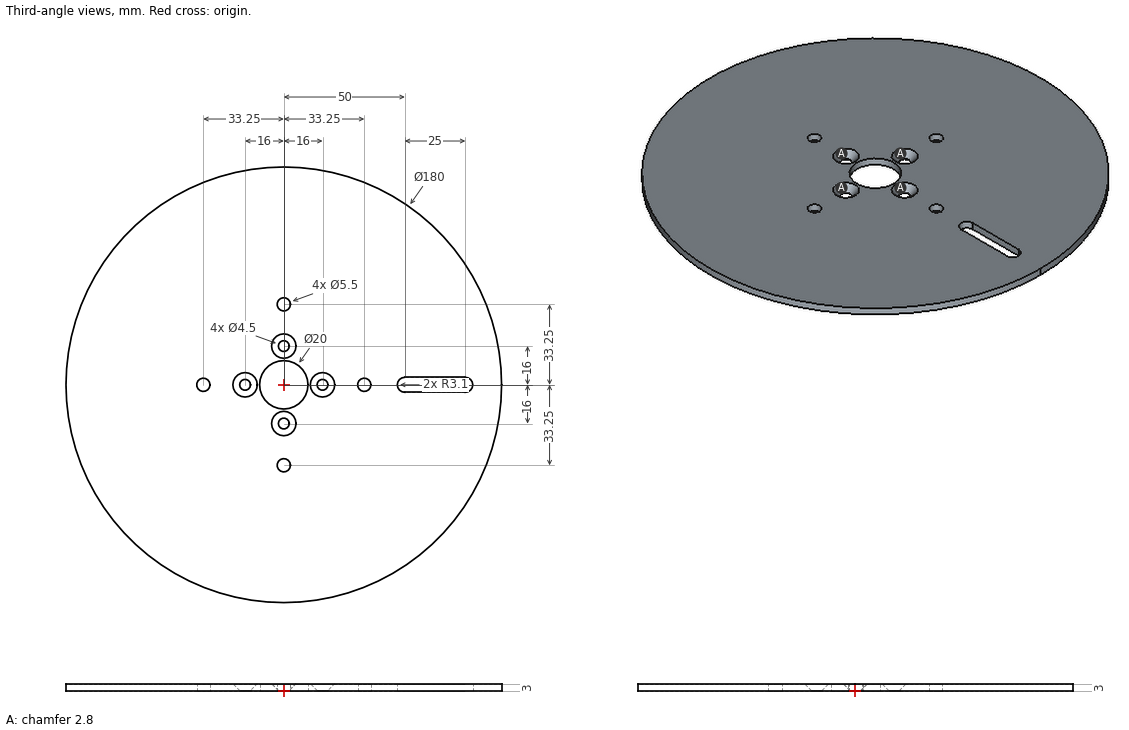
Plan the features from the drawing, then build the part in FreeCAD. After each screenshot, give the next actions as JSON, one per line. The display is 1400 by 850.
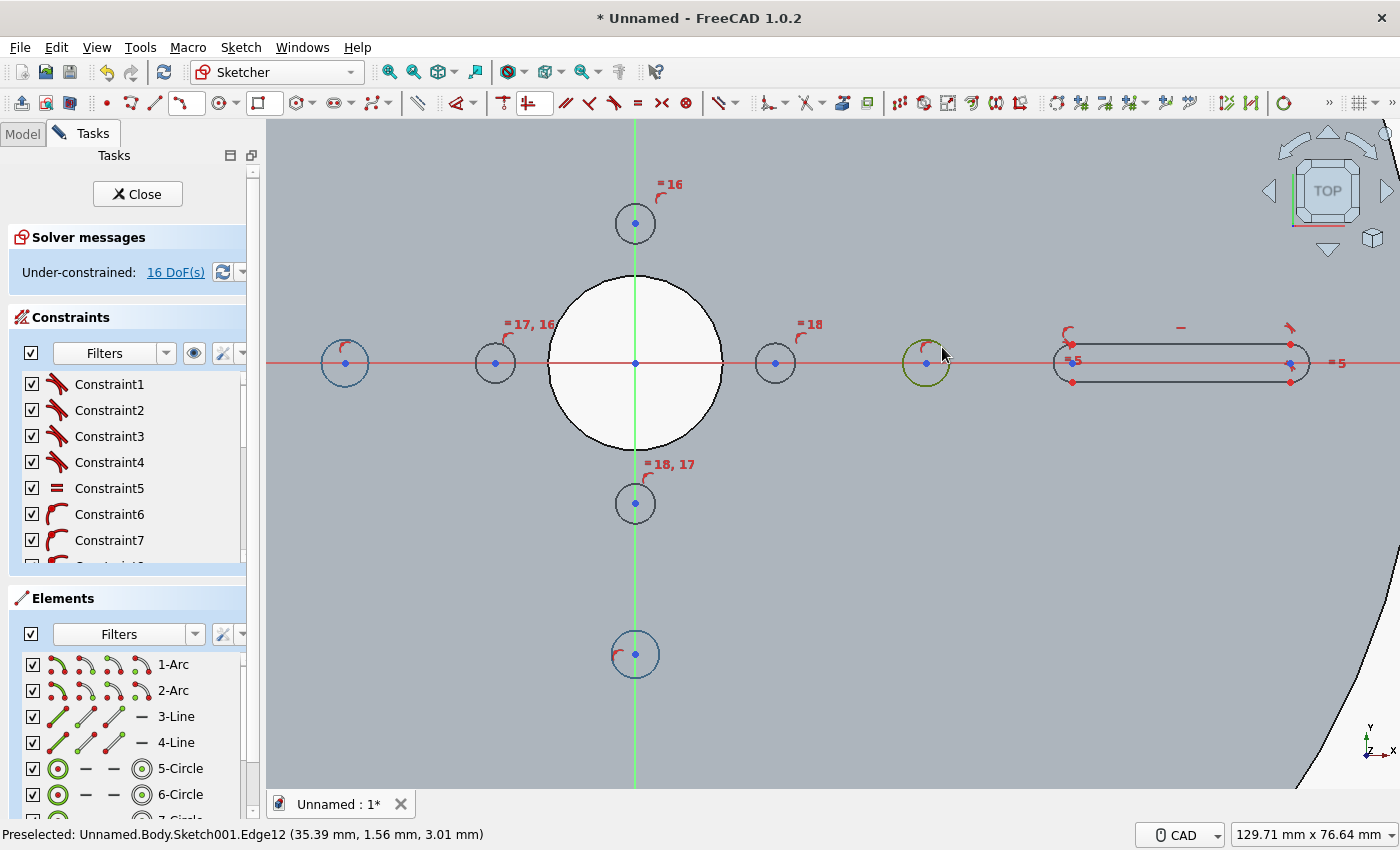
{"action": "left_click", "coordinate": [638, 104]}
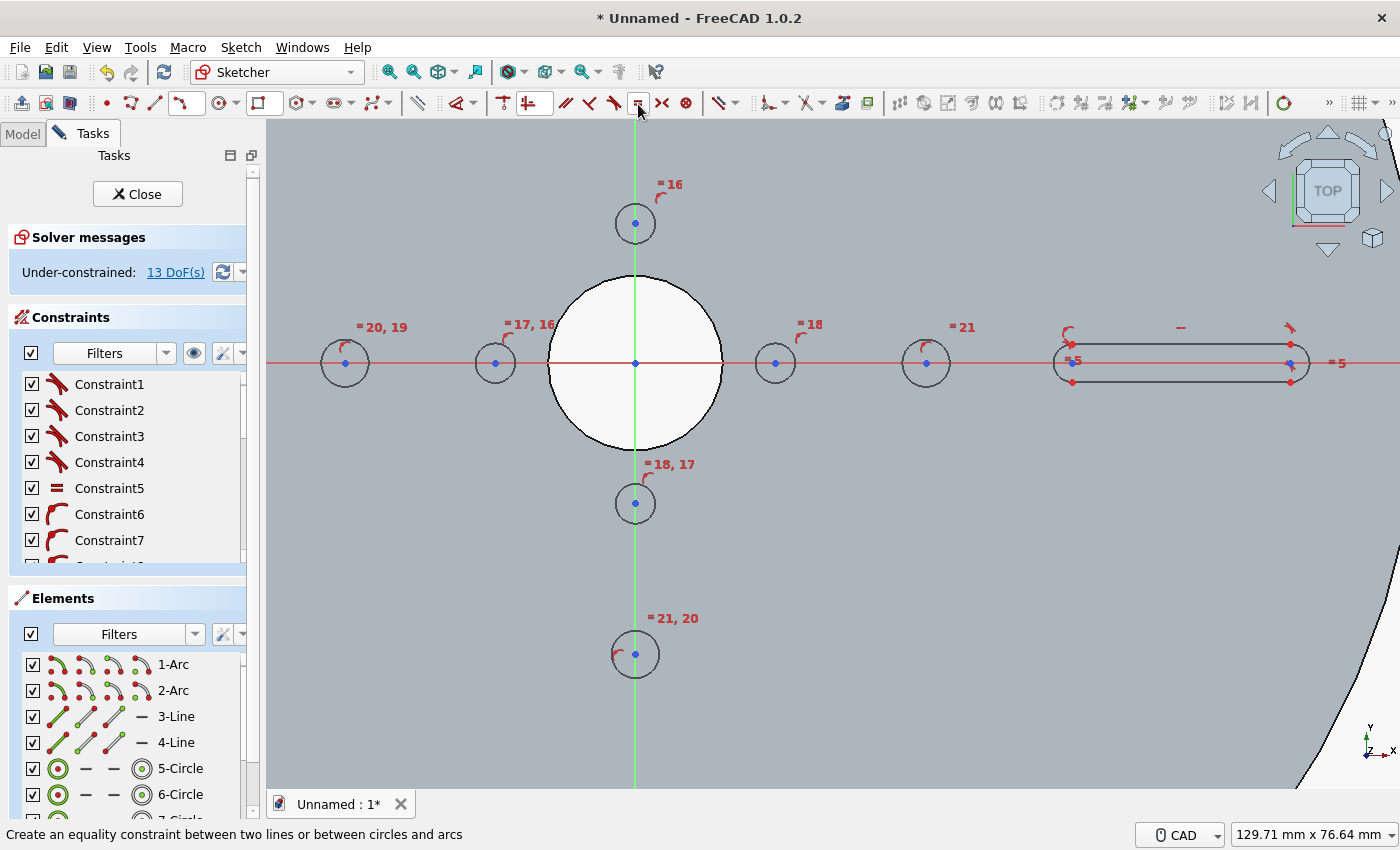
{"action": "left_click", "coordinate": [456, 104]}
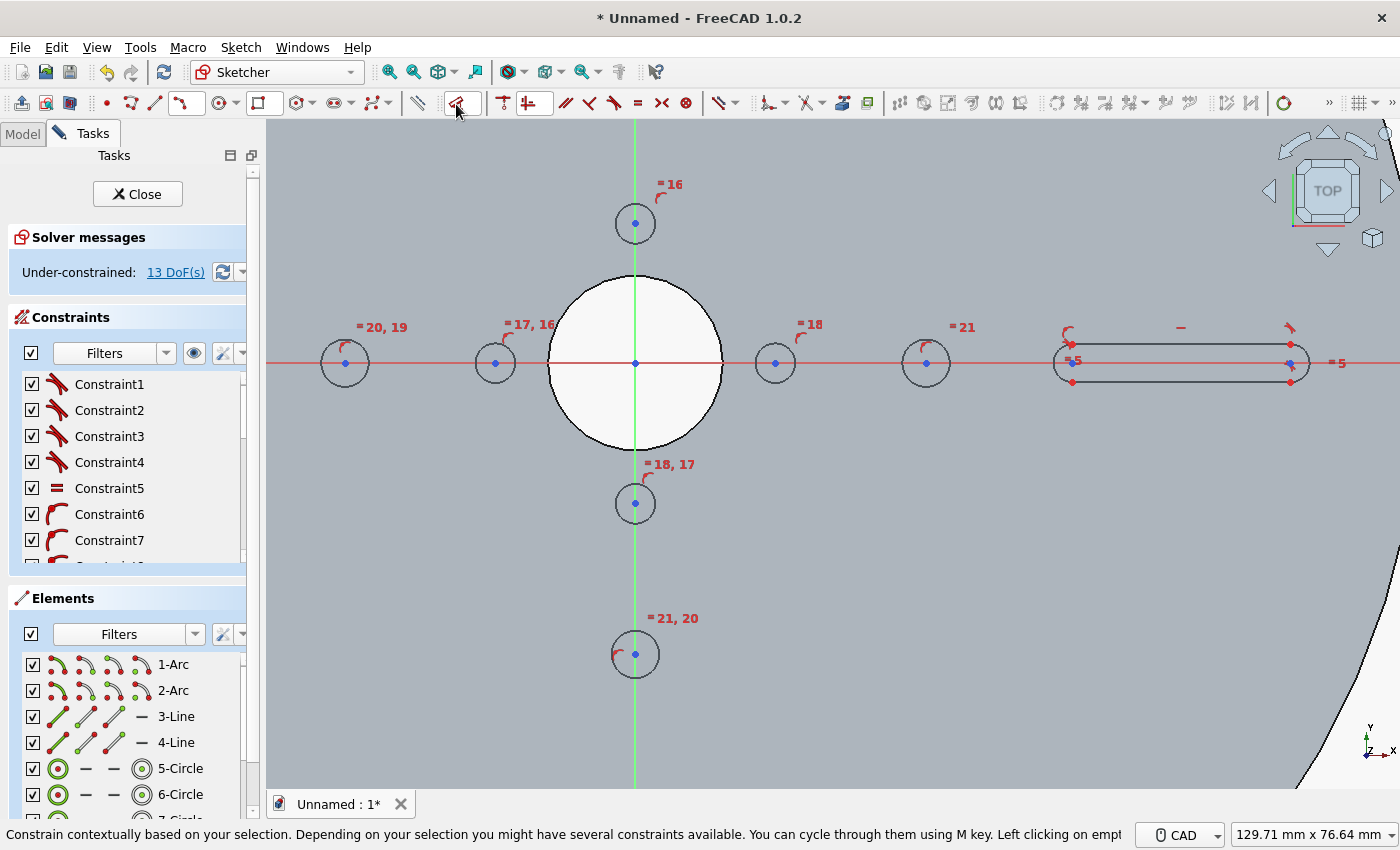
{"action": "scroll", "coordinate": [1057, 352], "scroll_direction": "up", "scroll_amount": 2}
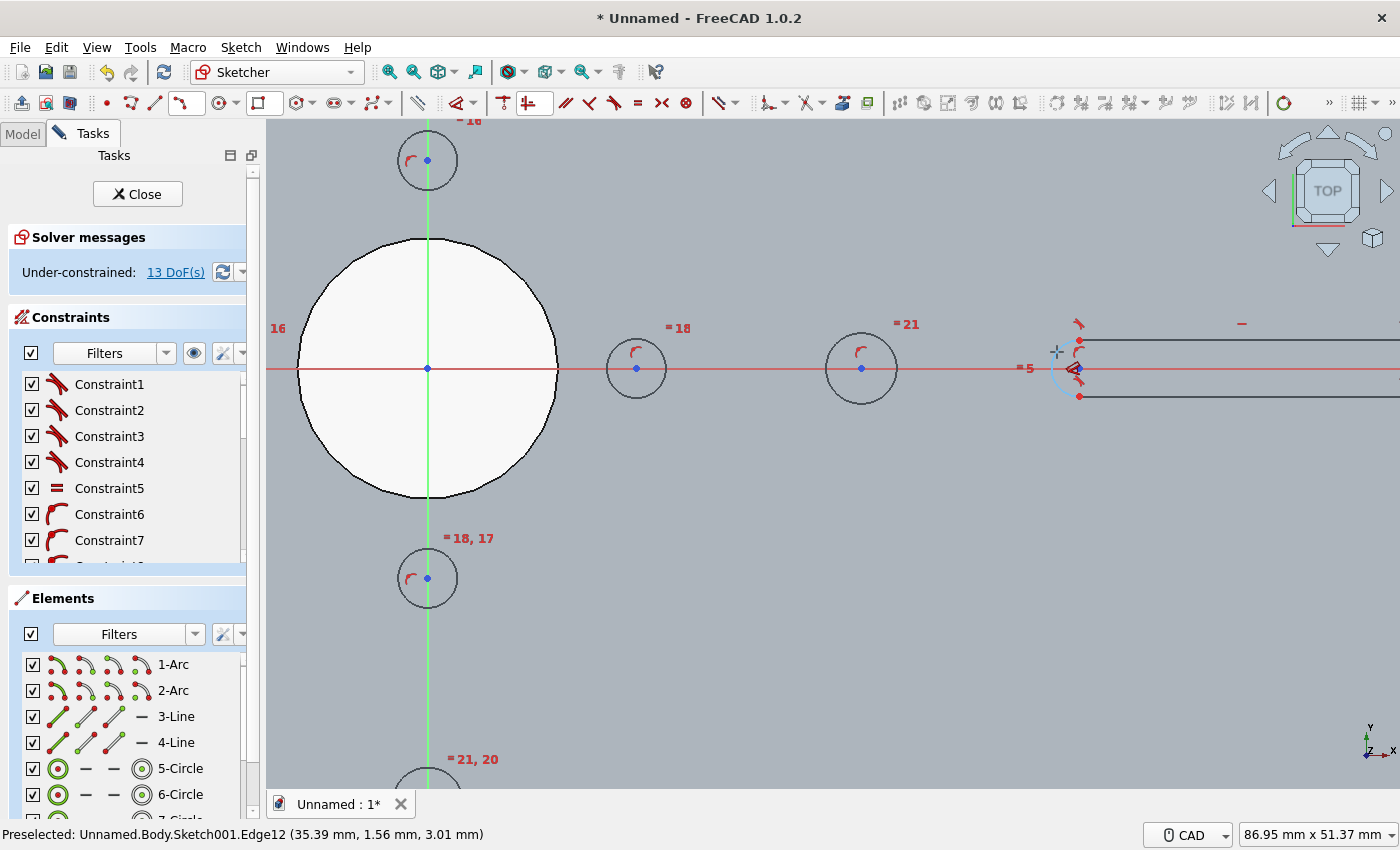
{"action": "left_click", "coordinate": [1057, 352]}
{"action": "left_click", "coordinate": [1031, 333]}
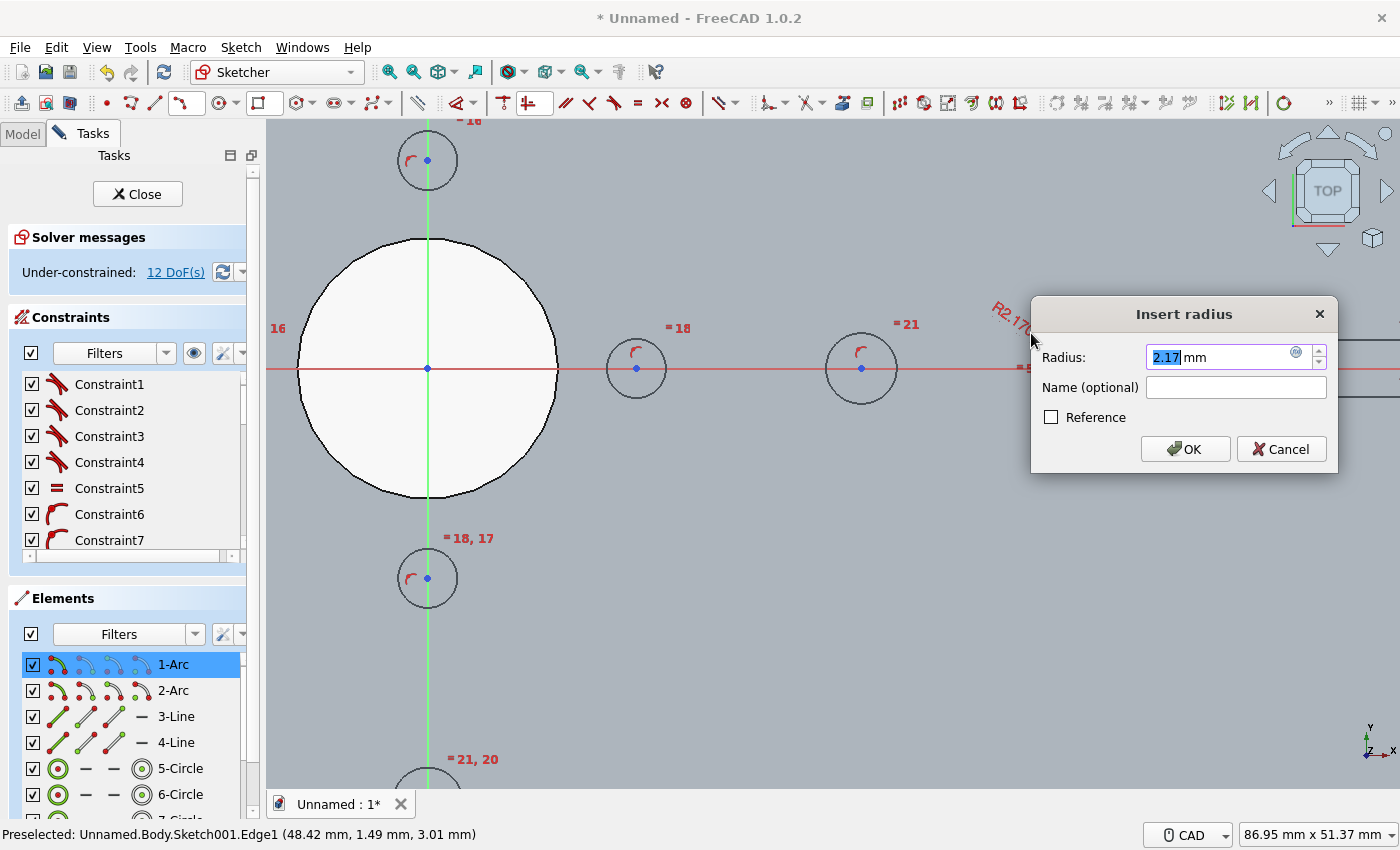
{"action": "type", "text": "3.1"}
{"action": "key", "text": "Return"}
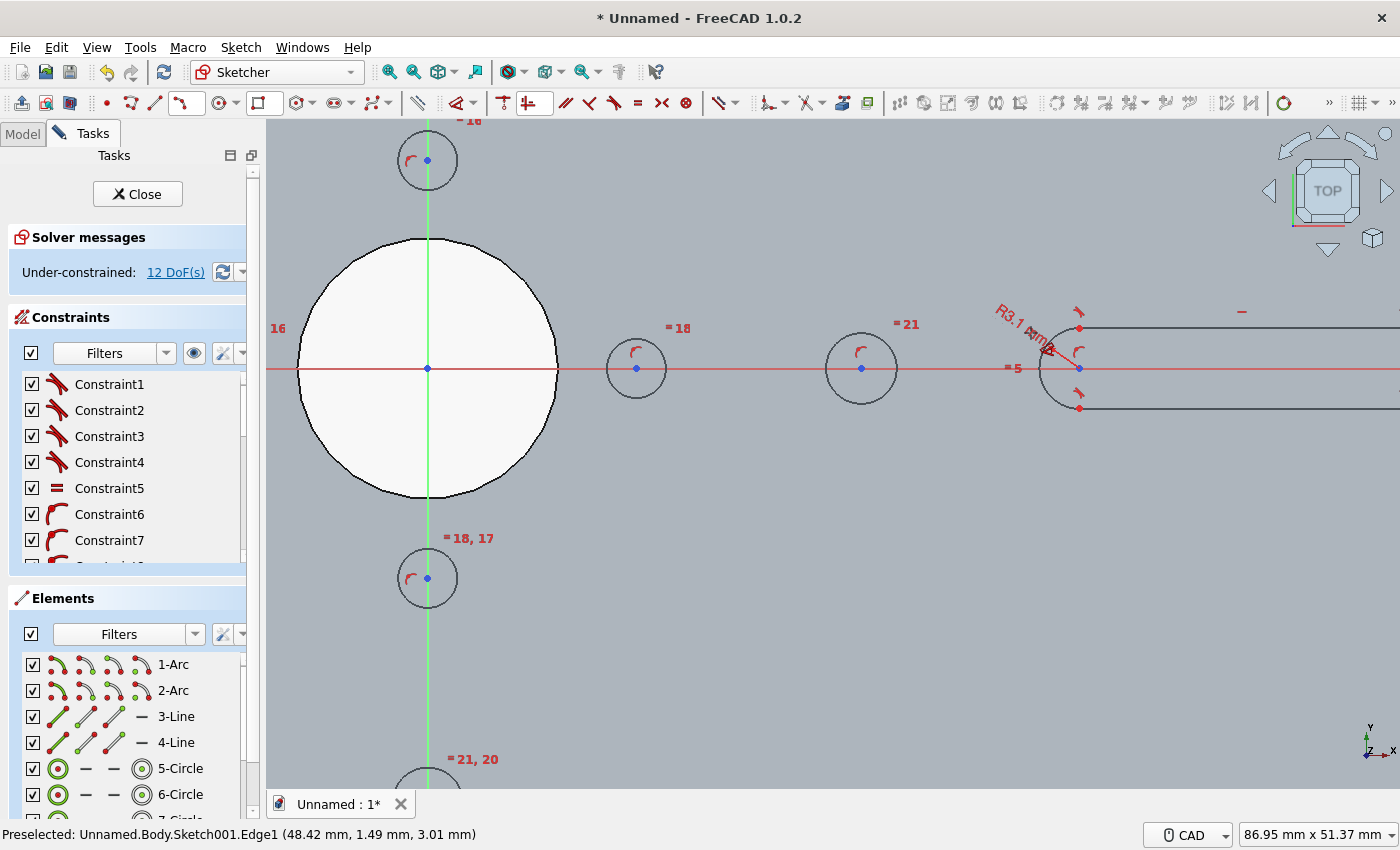
{"action": "left_click", "coordinate": [407, 182]}
{"action": "left_click", "coordinate": [385, 205]}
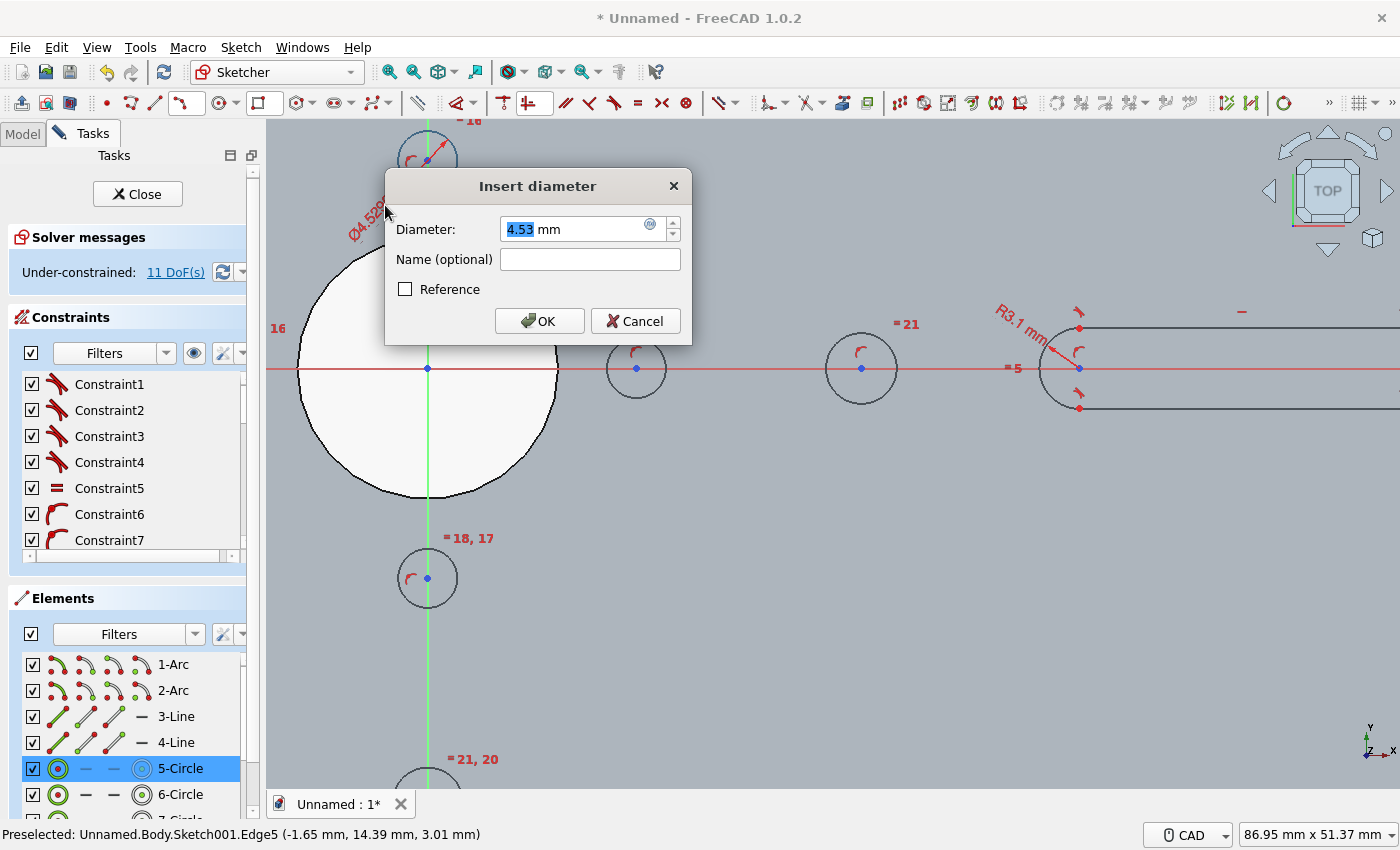
{"action": "type", "text": "4.5"}
{"action": "key", "text": "Return"}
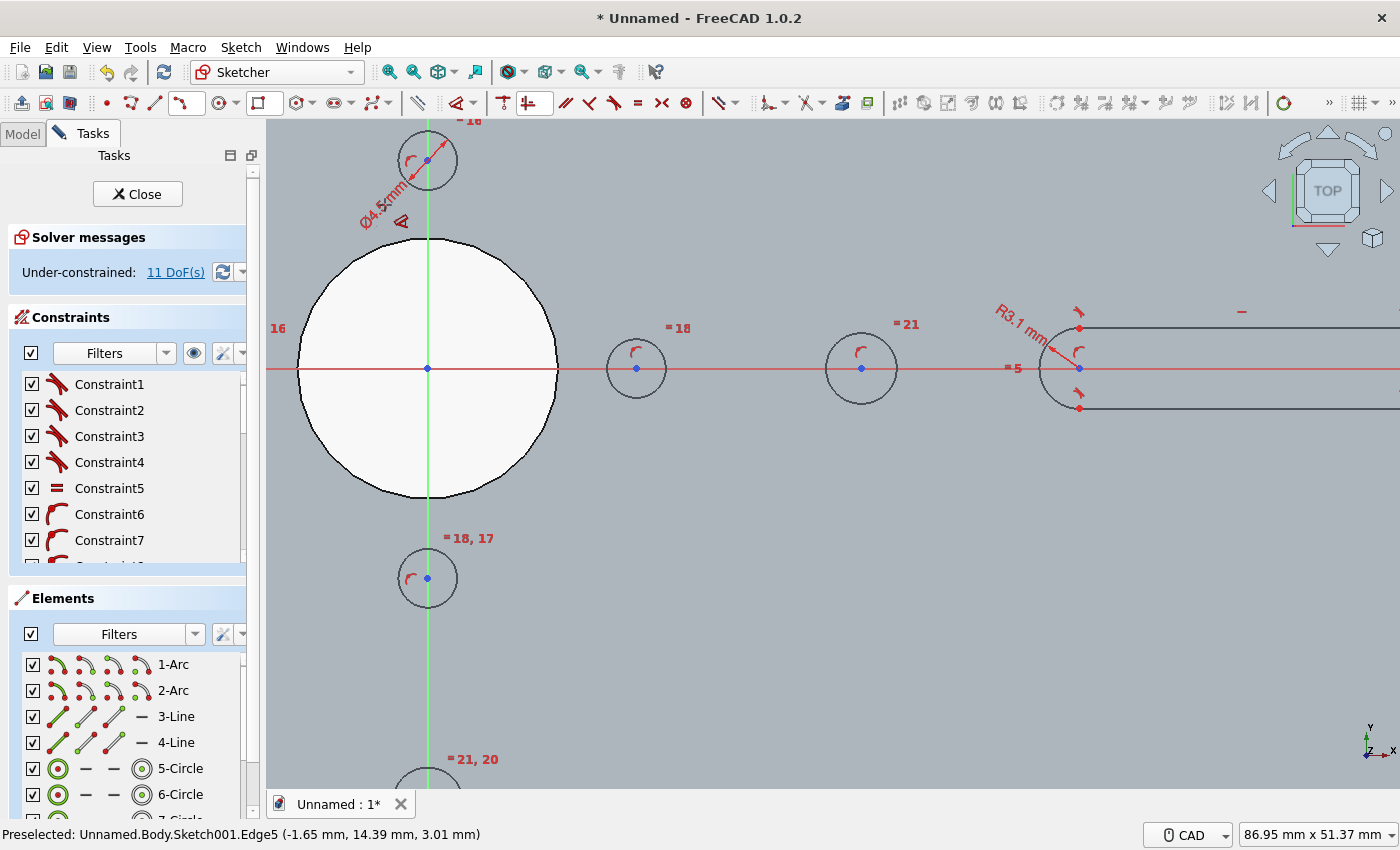
{"action": "scroll", "coordinate": [815, 524], "scroll_direction": "down", "scroll_amount": 4}